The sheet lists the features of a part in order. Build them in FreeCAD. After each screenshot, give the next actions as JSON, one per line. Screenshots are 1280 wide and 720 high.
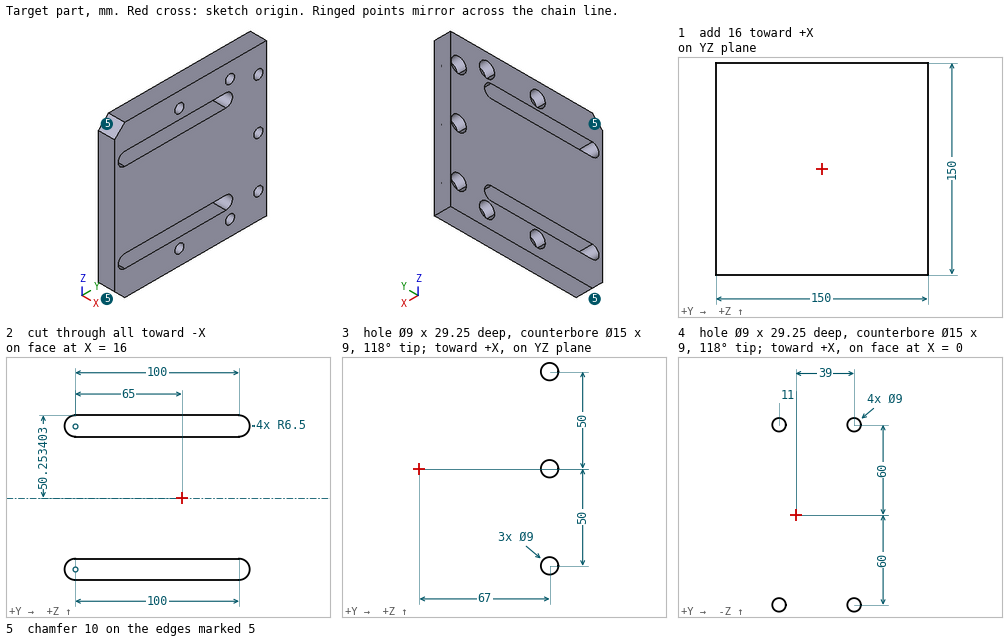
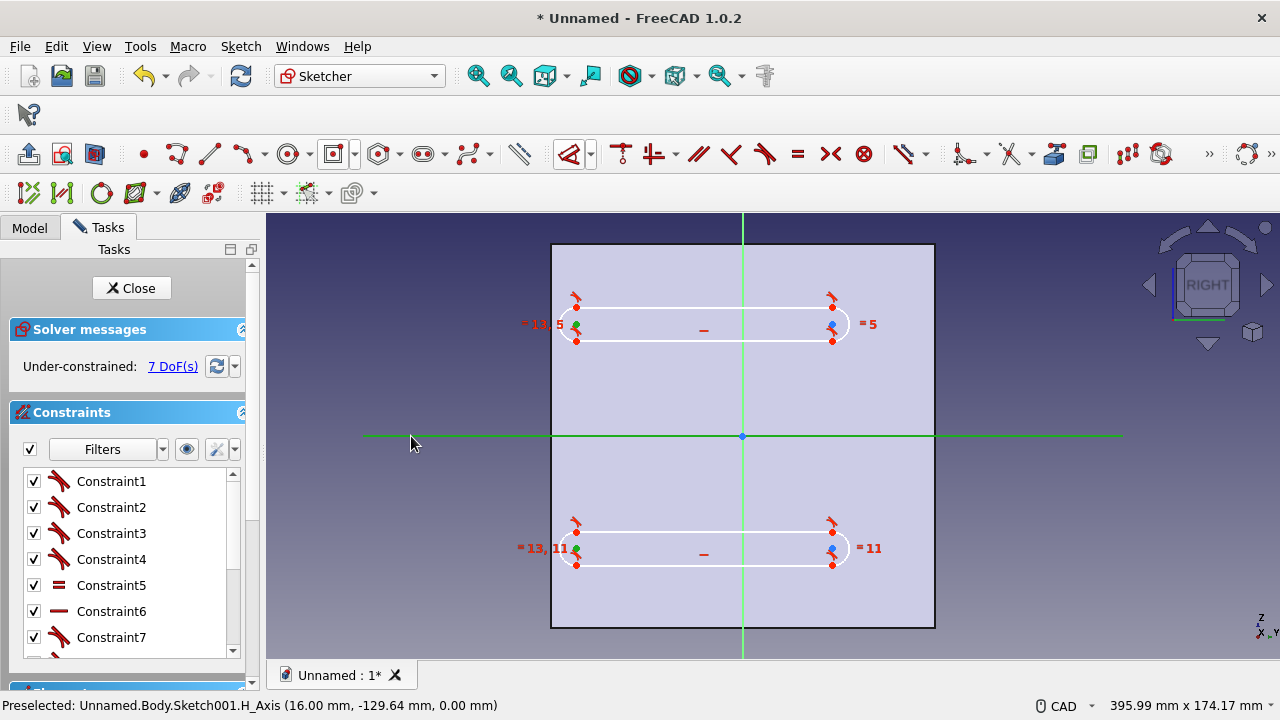
{"action": "left_click", "coordinate": [831, 154]}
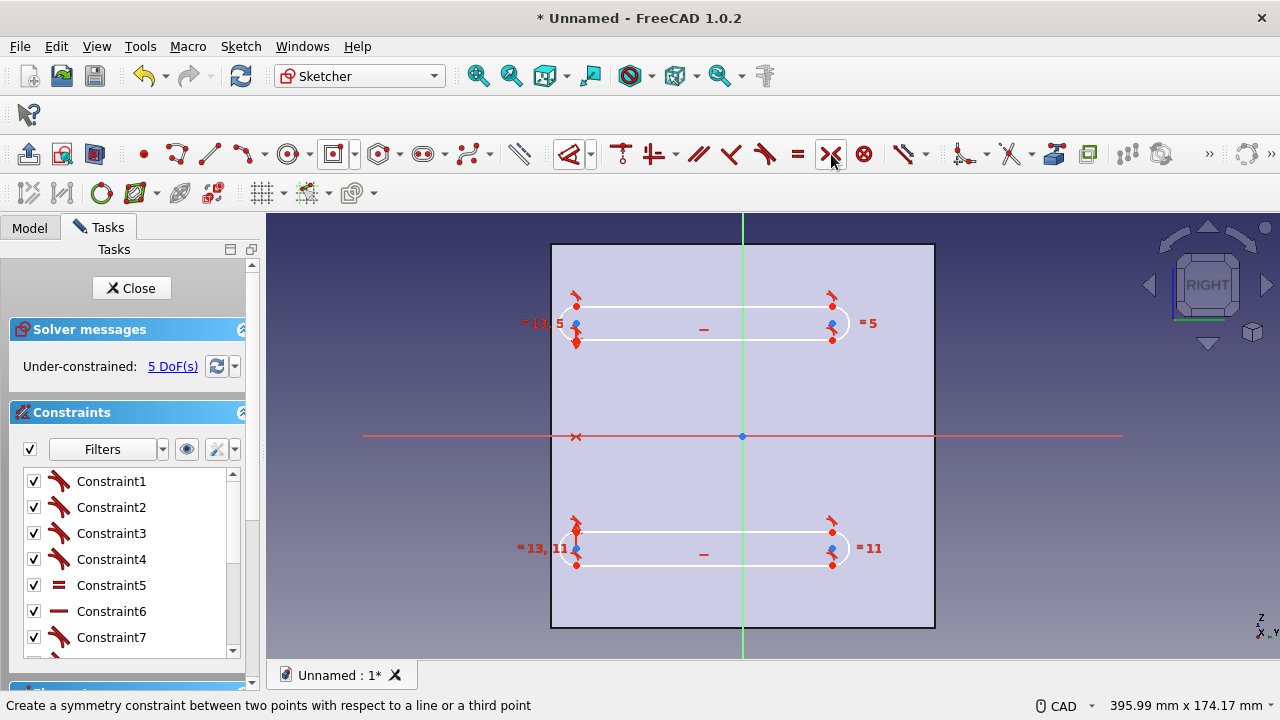
{"action": "left_click", "coordinate": [568, 154]}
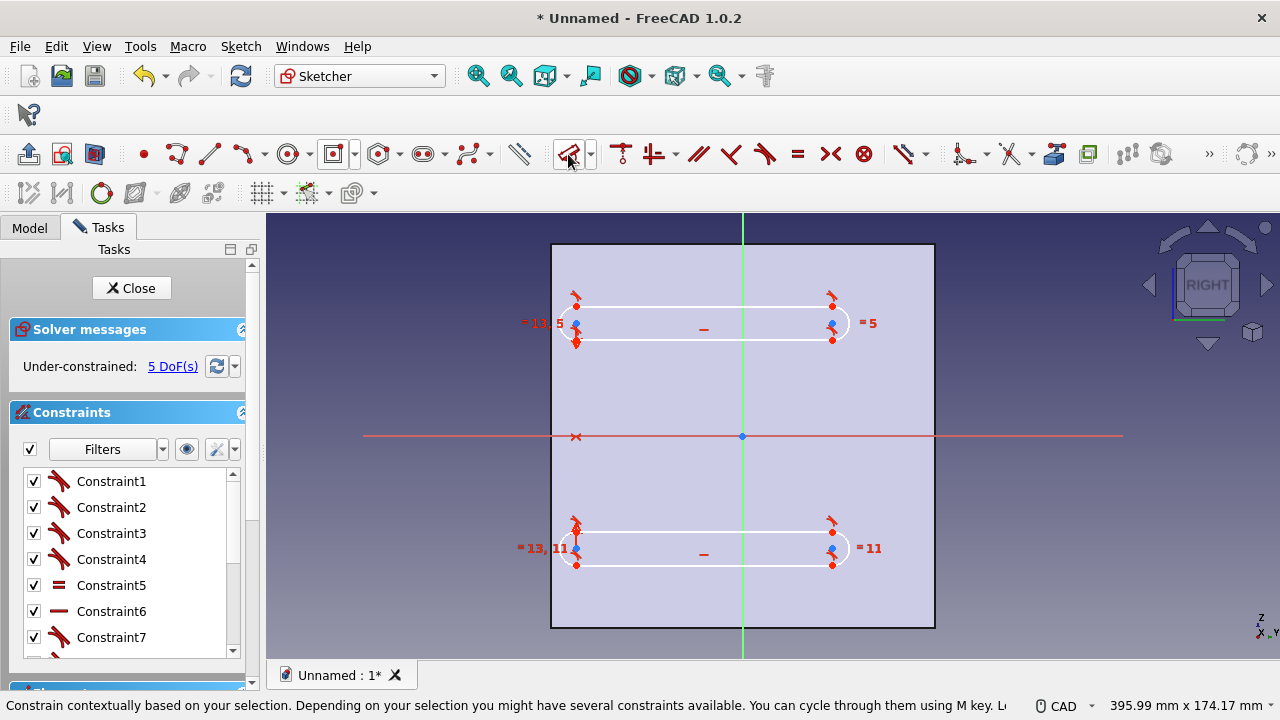
{"action": "scroll", "coordinate": [563, 314], "scroll_direction": "up", "scroll_amount": 5}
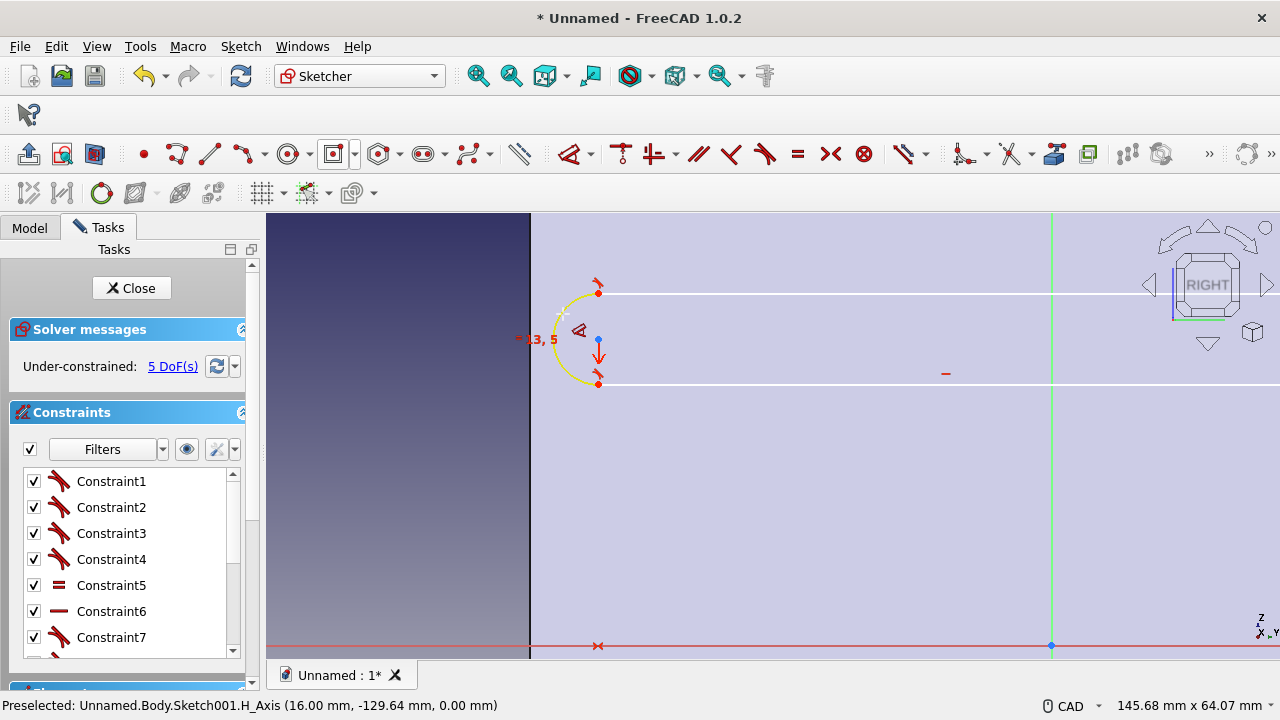
{"action": "left_click", "coordinate": [562, 313]}
{"action": "left_click", "coordinate": [536, 294]}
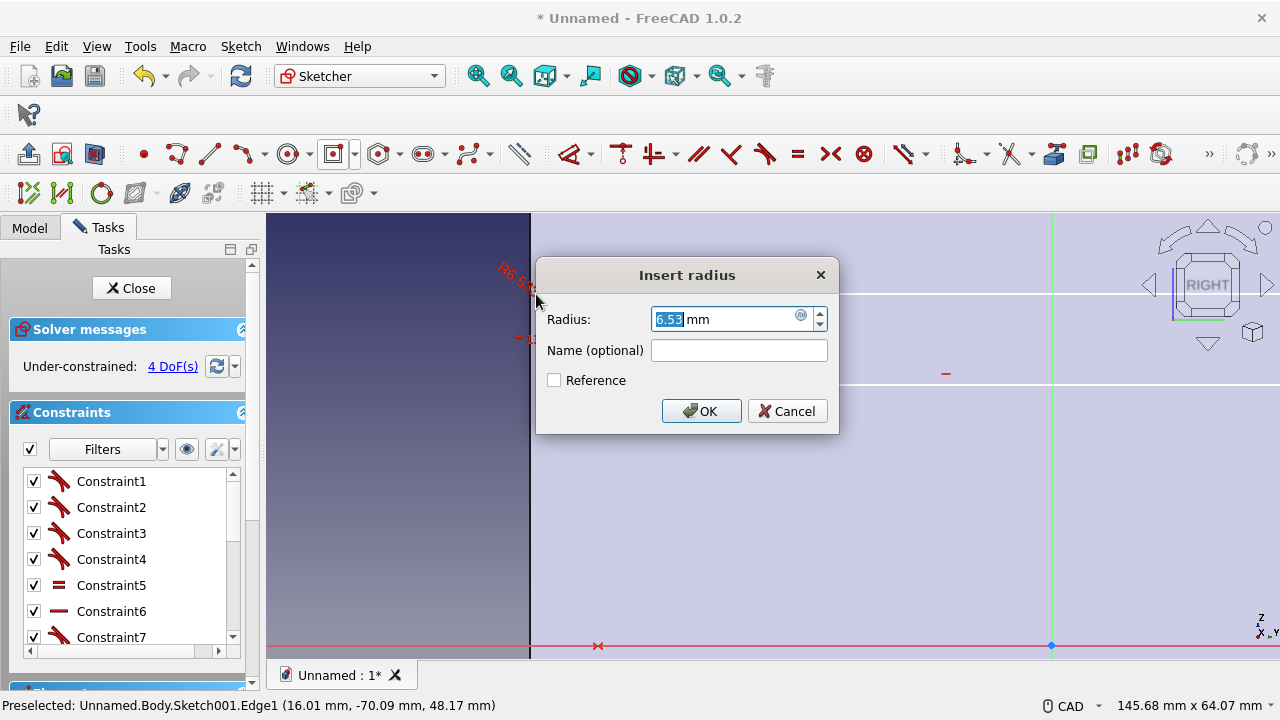
{"action": "type", "text": "6.5"}
{"action": "key", "text": "Return"}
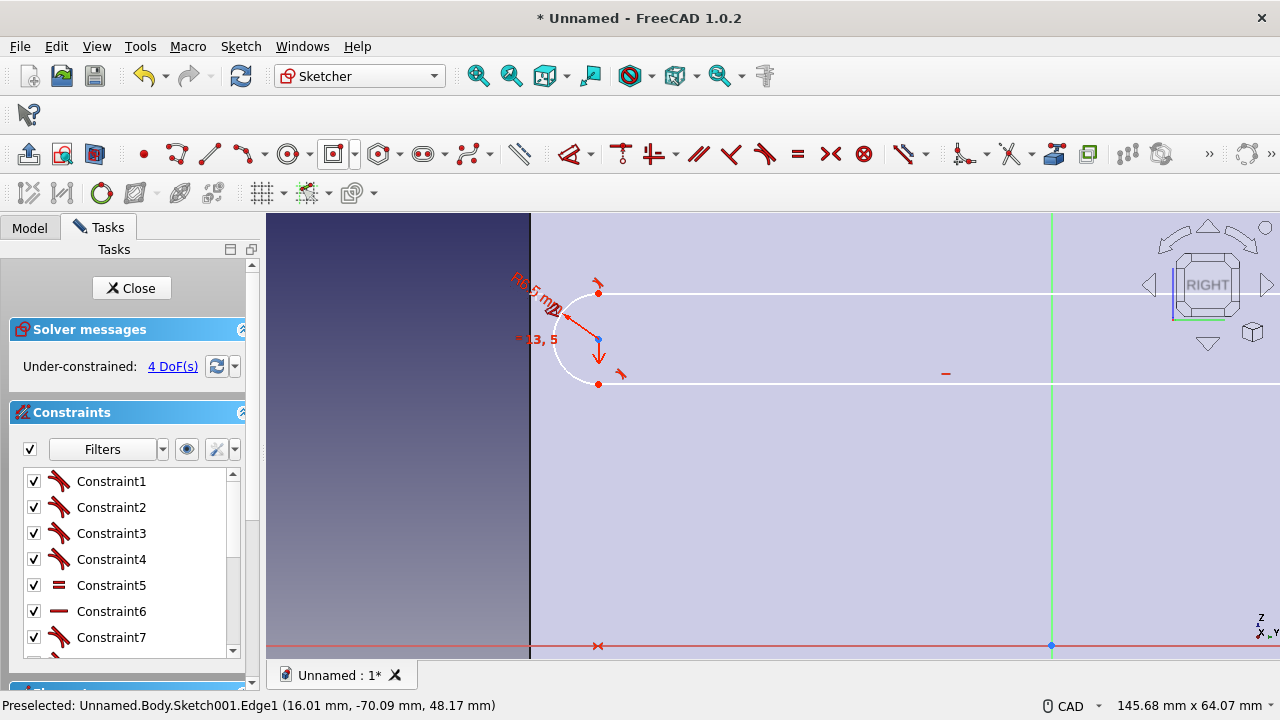
{"action": "left_click", "coordinate": [808, 294]}
{"action": "left_click", "coordinate": [857, 260]}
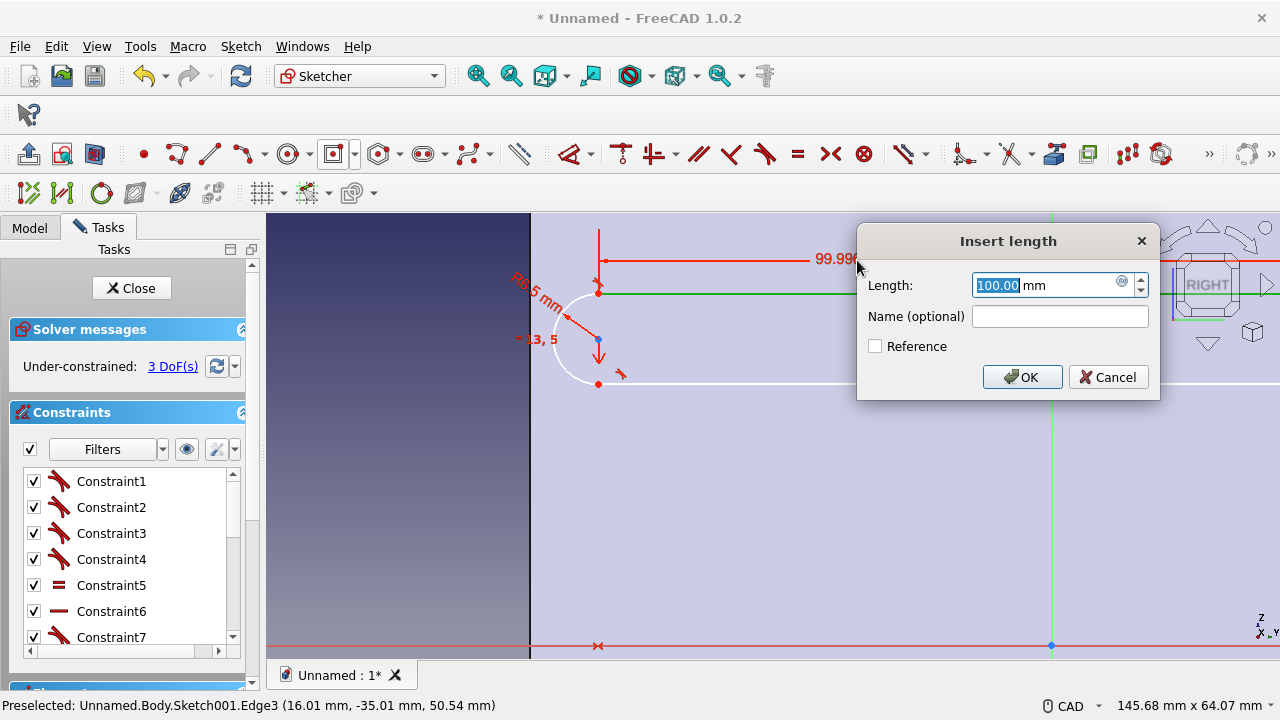
{"action": "type", "text": "100"}
{"action": "key", "text": "Return"}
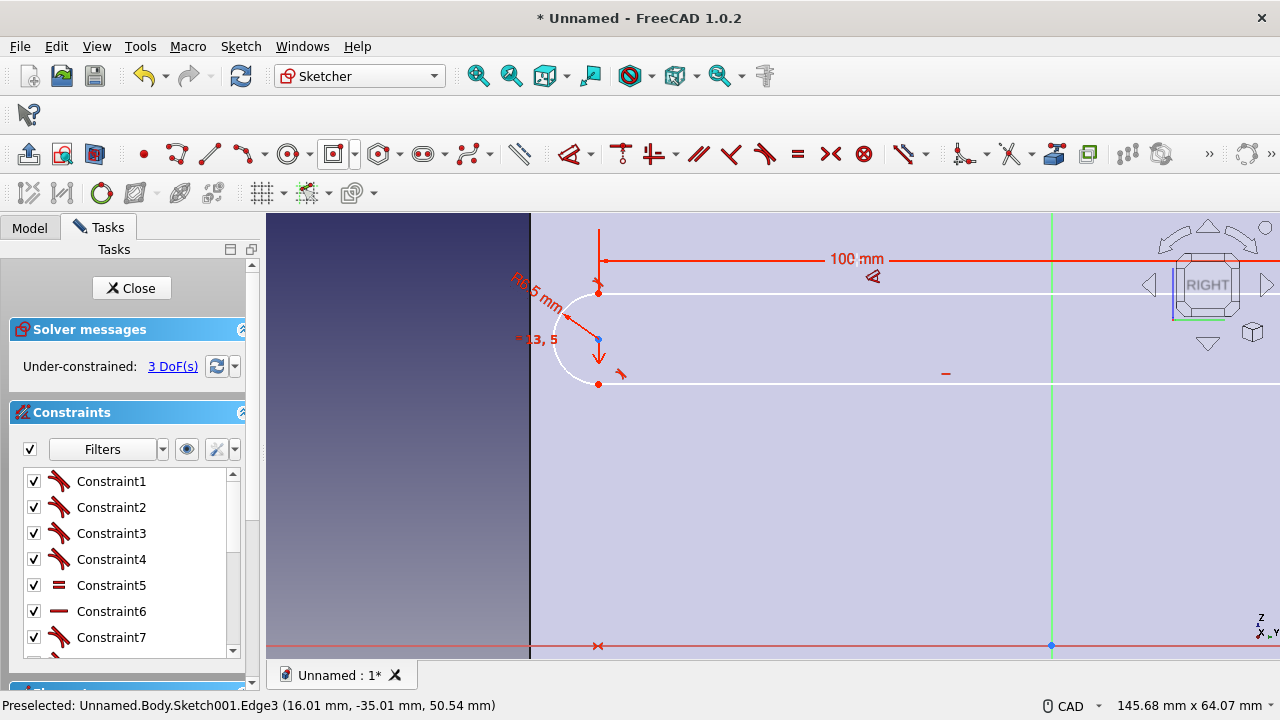
{"action": "scroll", "coordinate": [563, 314], "scroll_direction": "down", "scroll_amount": 5}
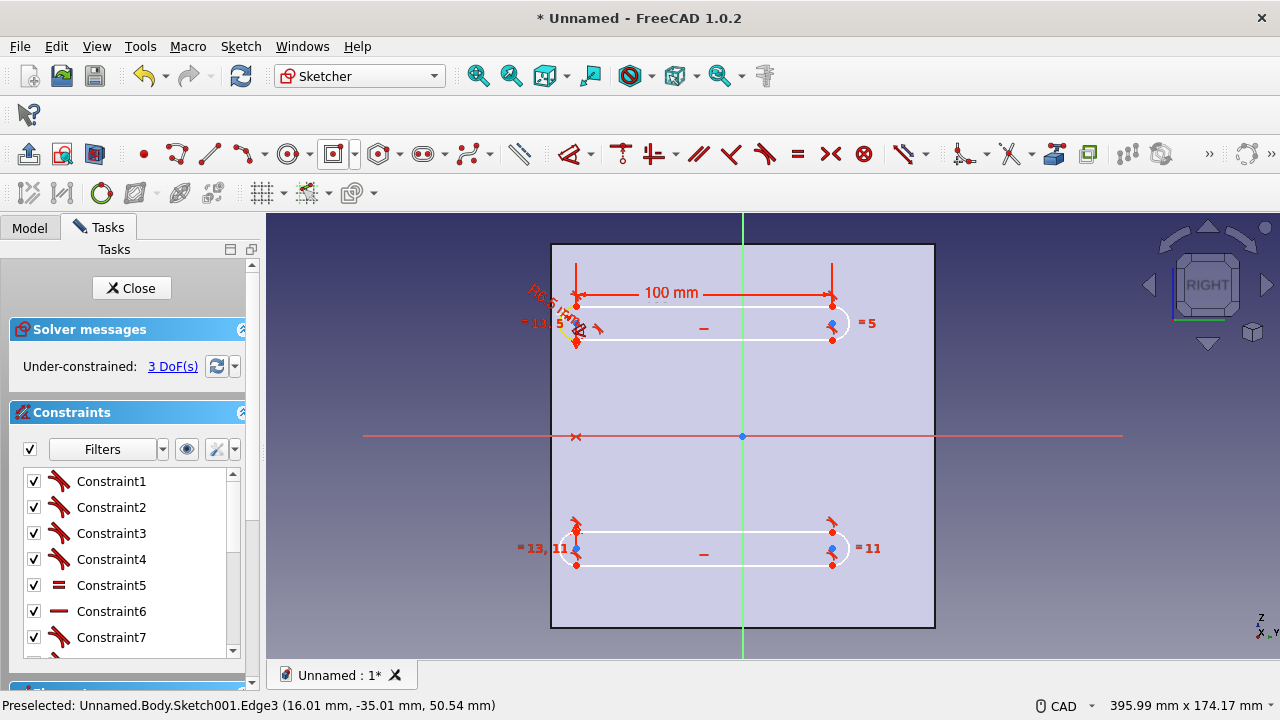
{"action": "left_click", "coordinate": [653, 532]}
{"action": "left_click", "coordinate": [704, 498]}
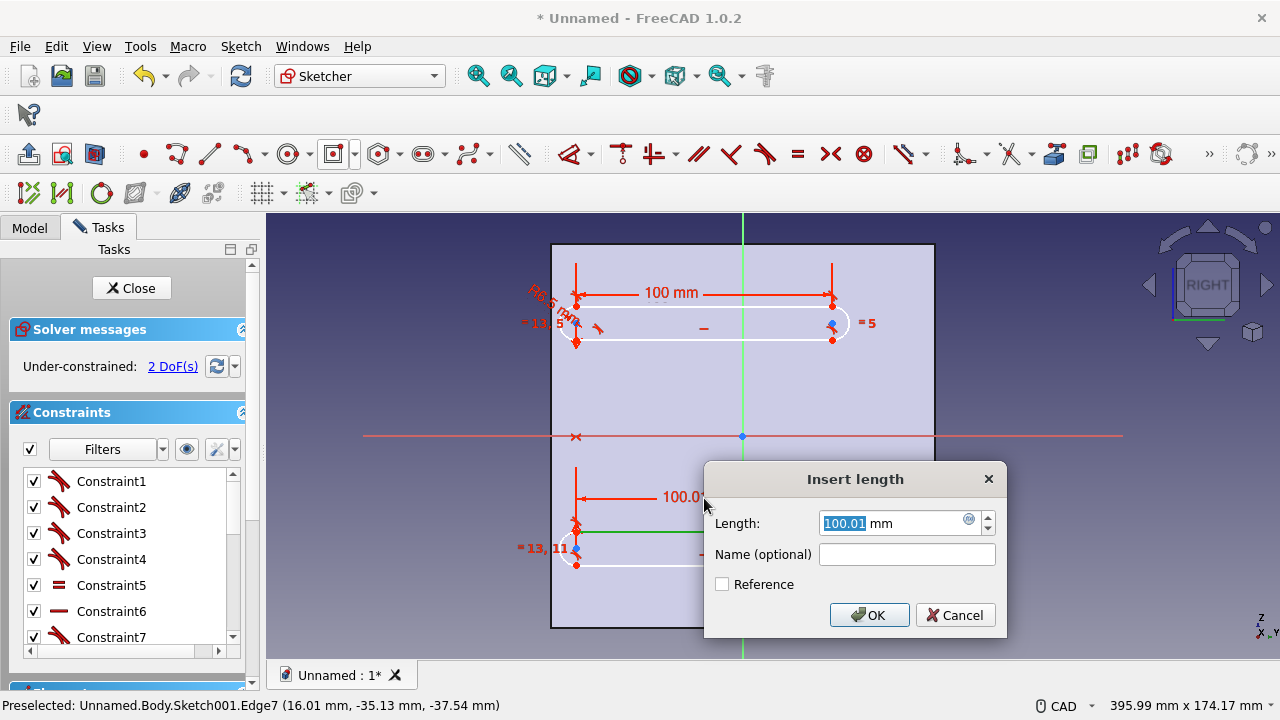
{"action": "type", "text": "100"}
{"action": "key", "text": "Return"}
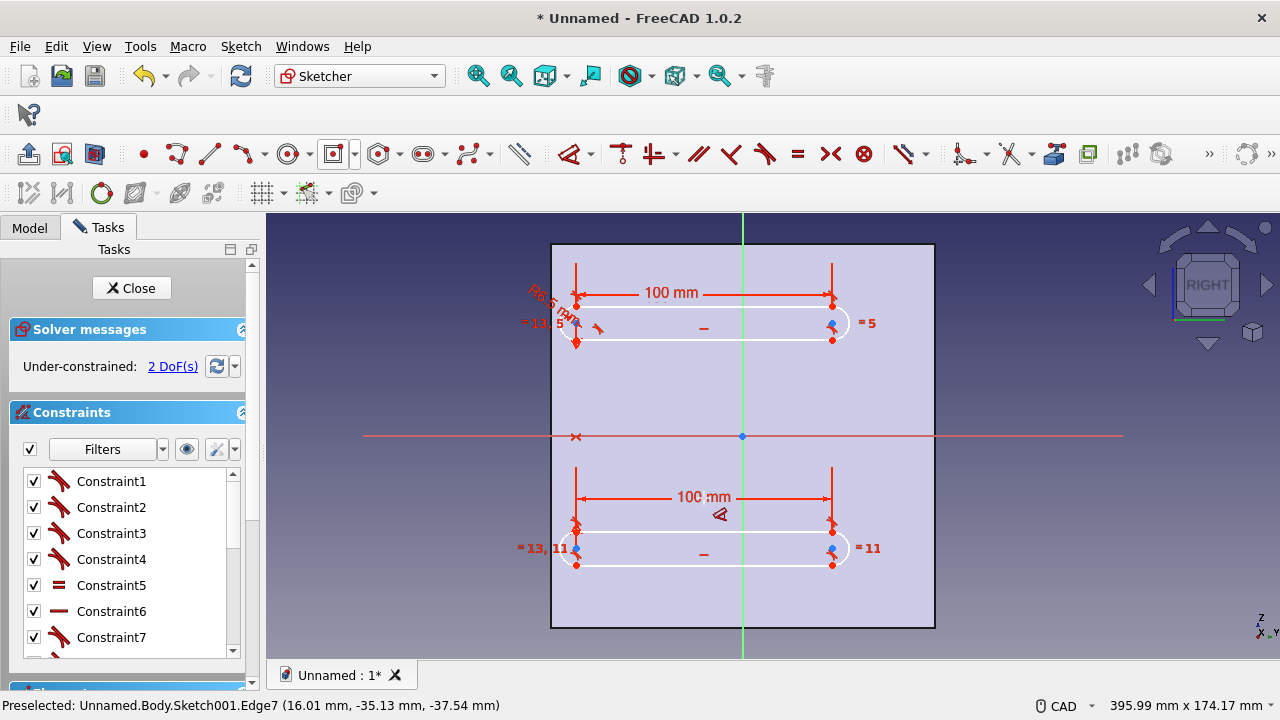
{"action": "left_click", "coordinate": [576, 307]}
{"action": "left_click", "coordinate": [660, 273]}